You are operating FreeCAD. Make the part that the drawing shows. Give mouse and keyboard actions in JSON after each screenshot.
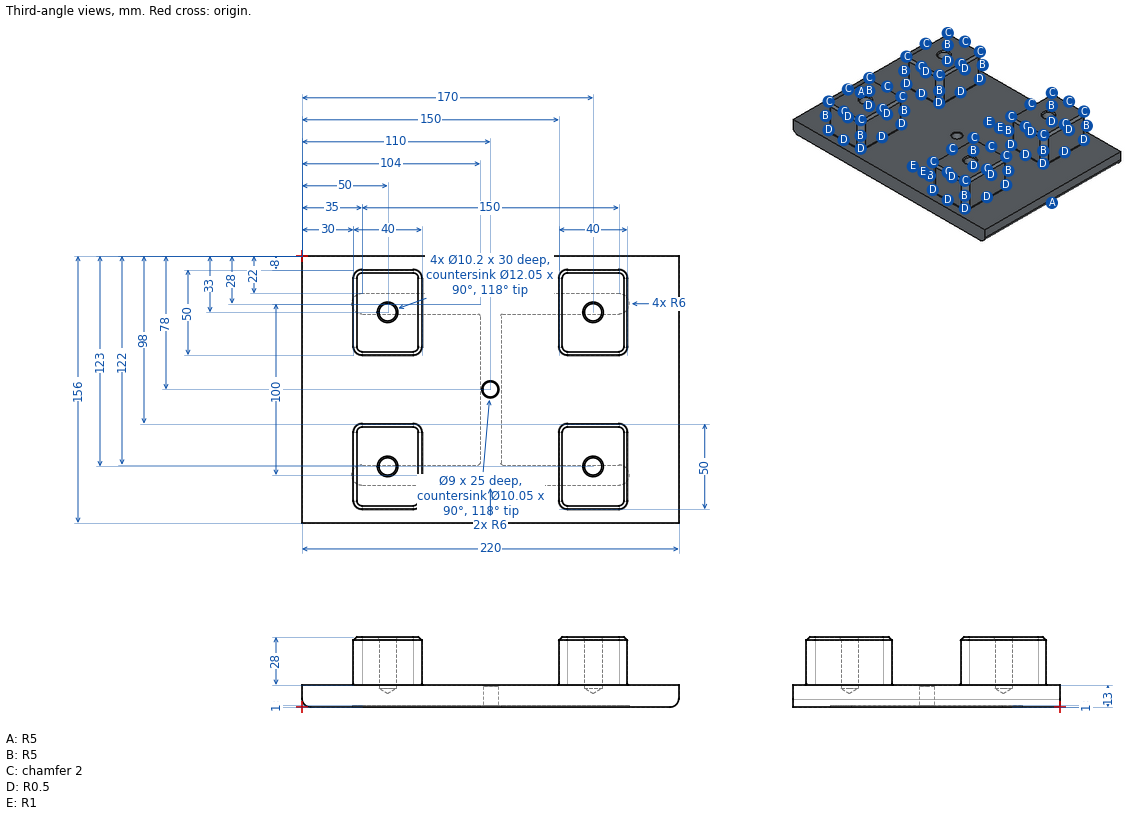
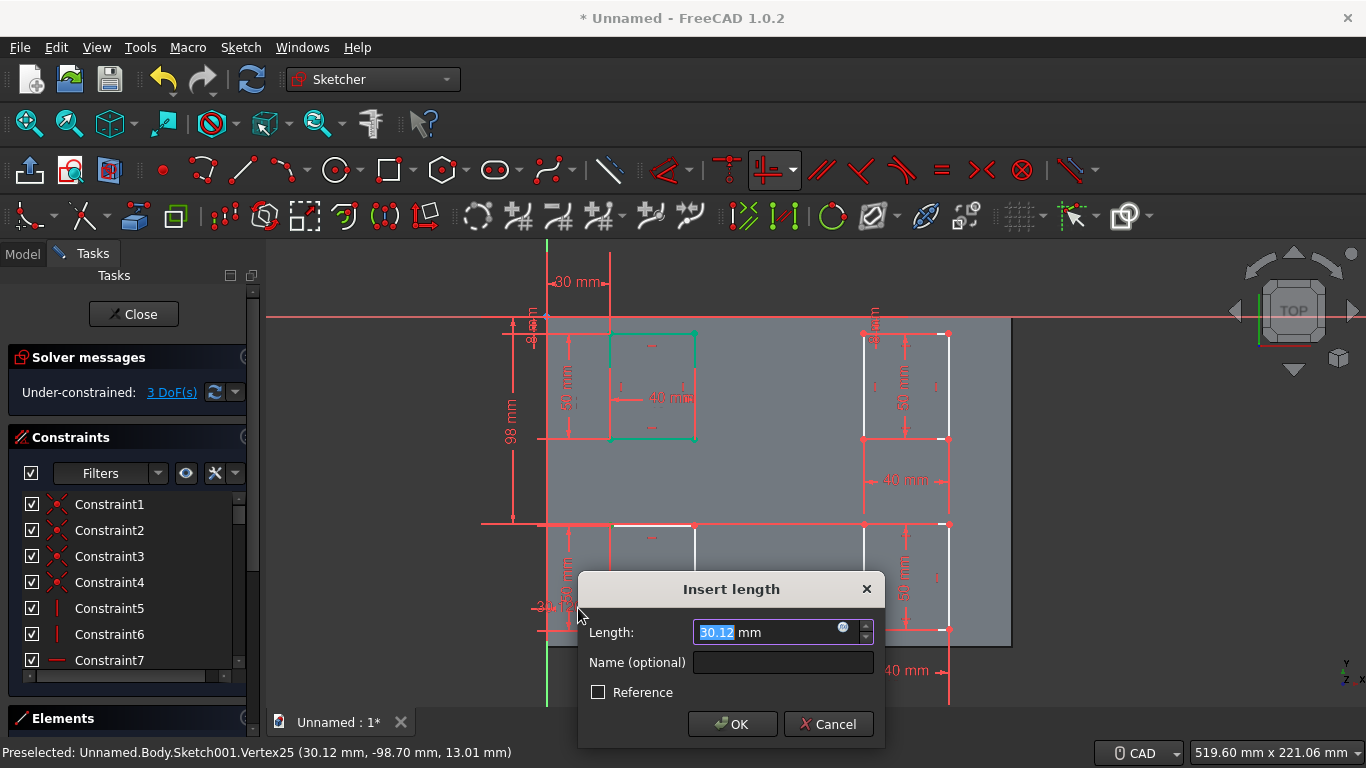
{"action": "type", "text": "30"}
{"action": "key", "text": "Return"}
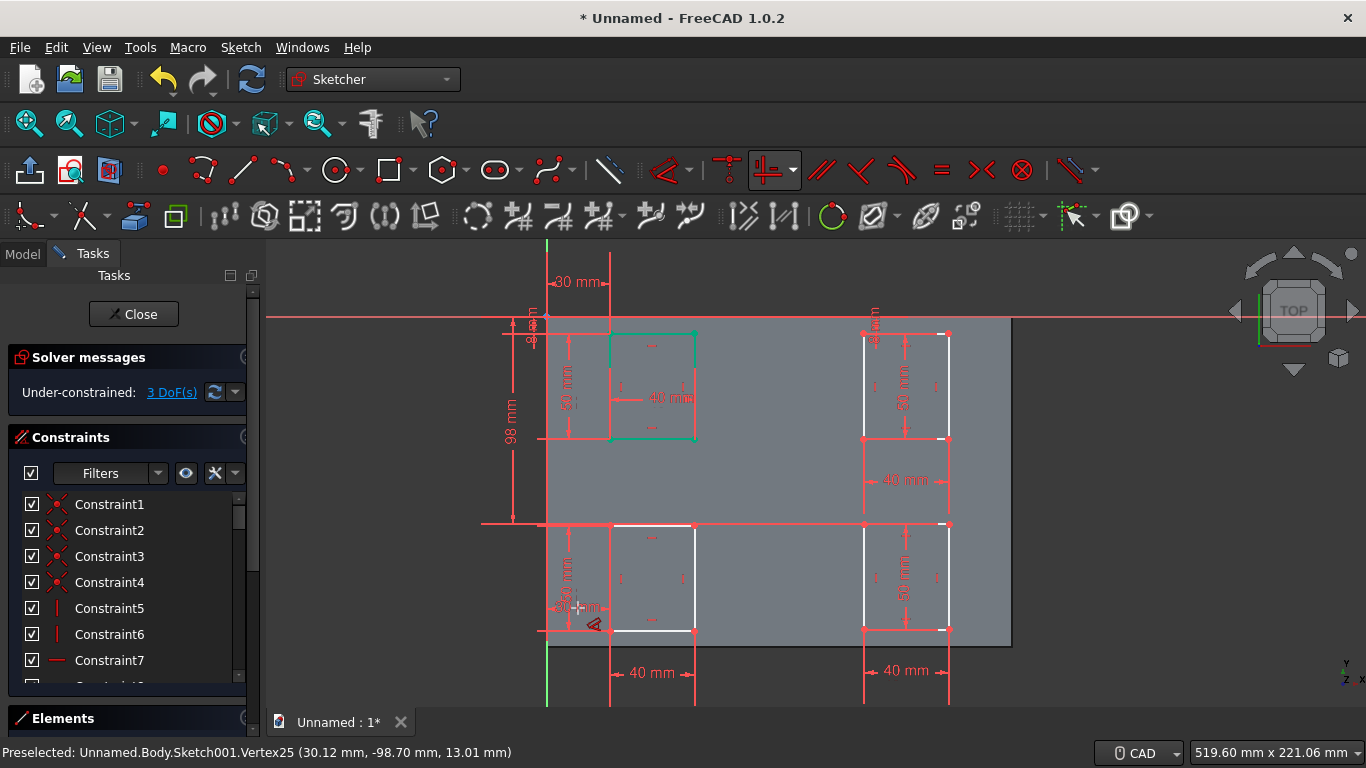
{"action": "left_click", "coordinate": [610, 526]}
{"action": "left_click", "coordinate": [513, 469]}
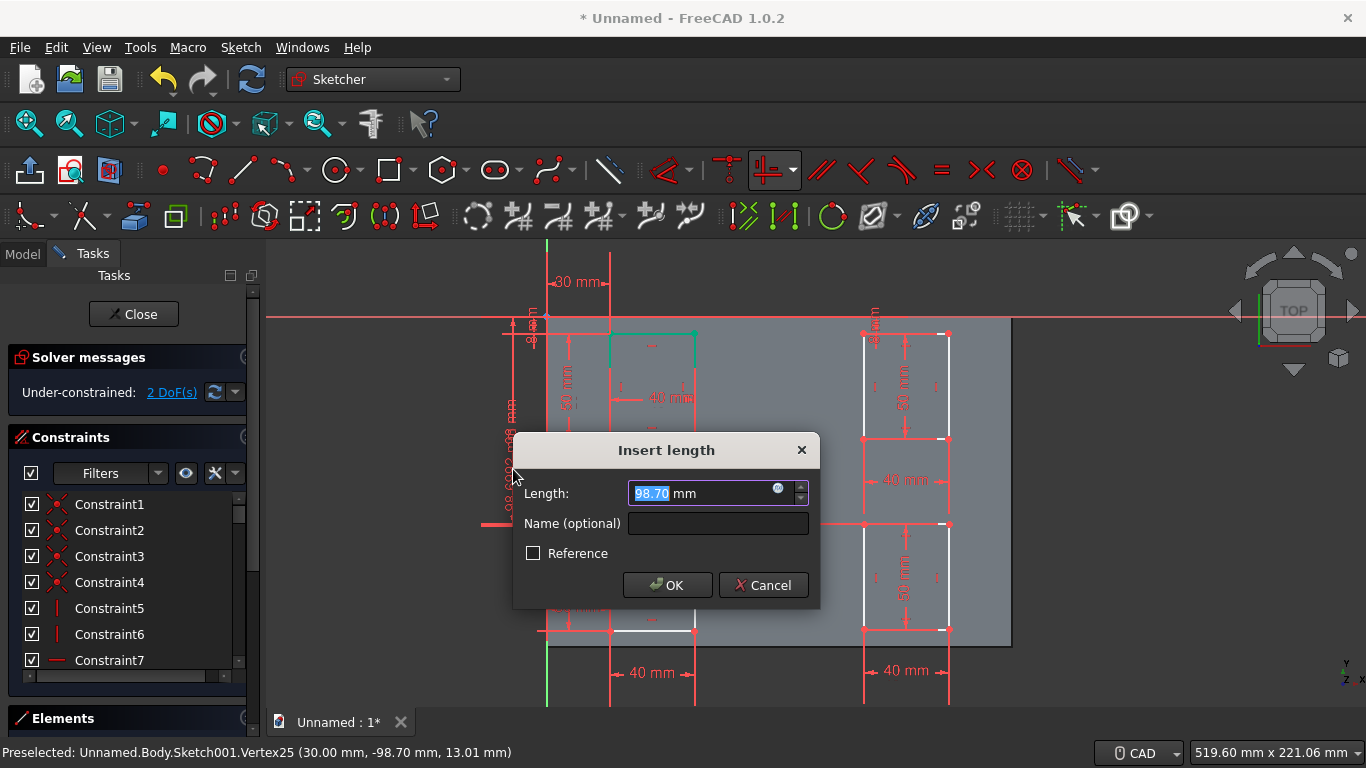
{"action": "type", "text": "98"}
{"action": "key", "text": "Return"}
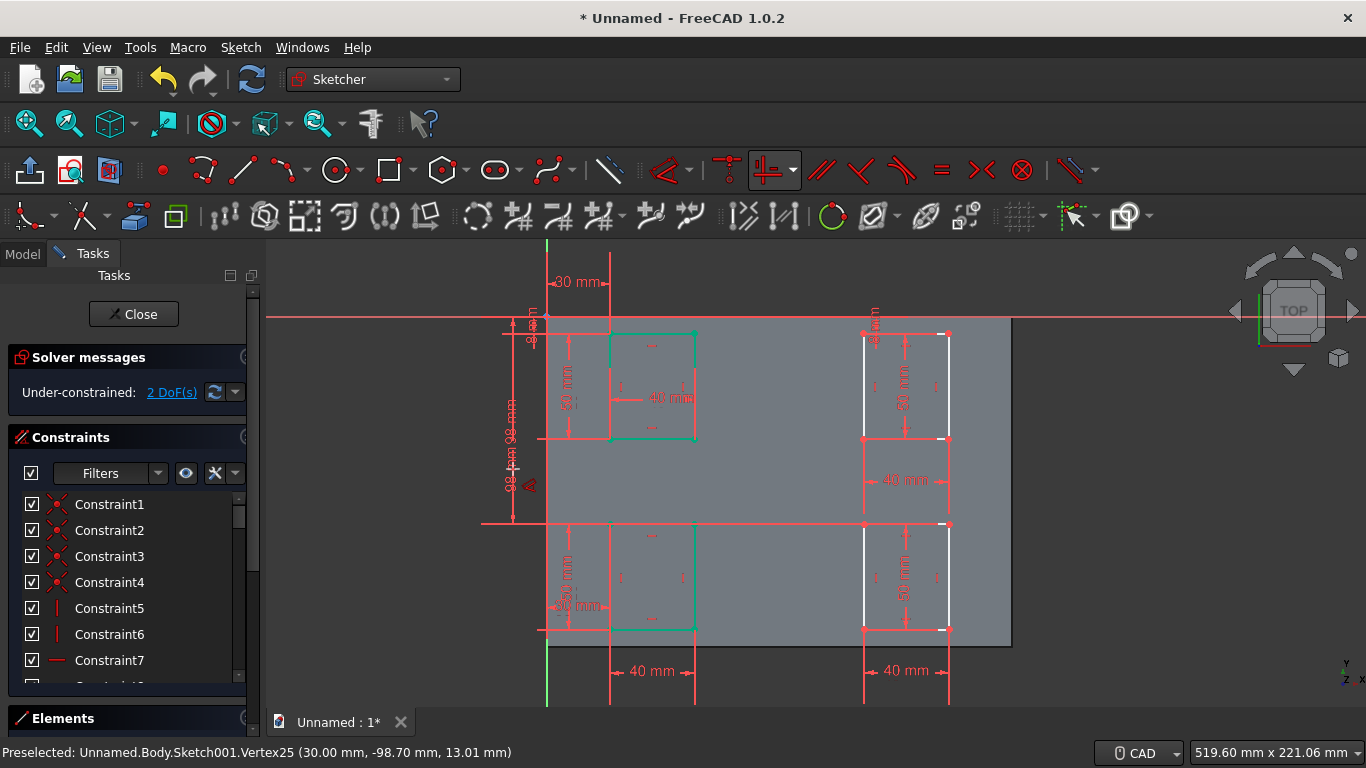
{"action": "left_click", "coordinate": [864, 334]}
{"action": "left_click", "coordinate": [705, 283]}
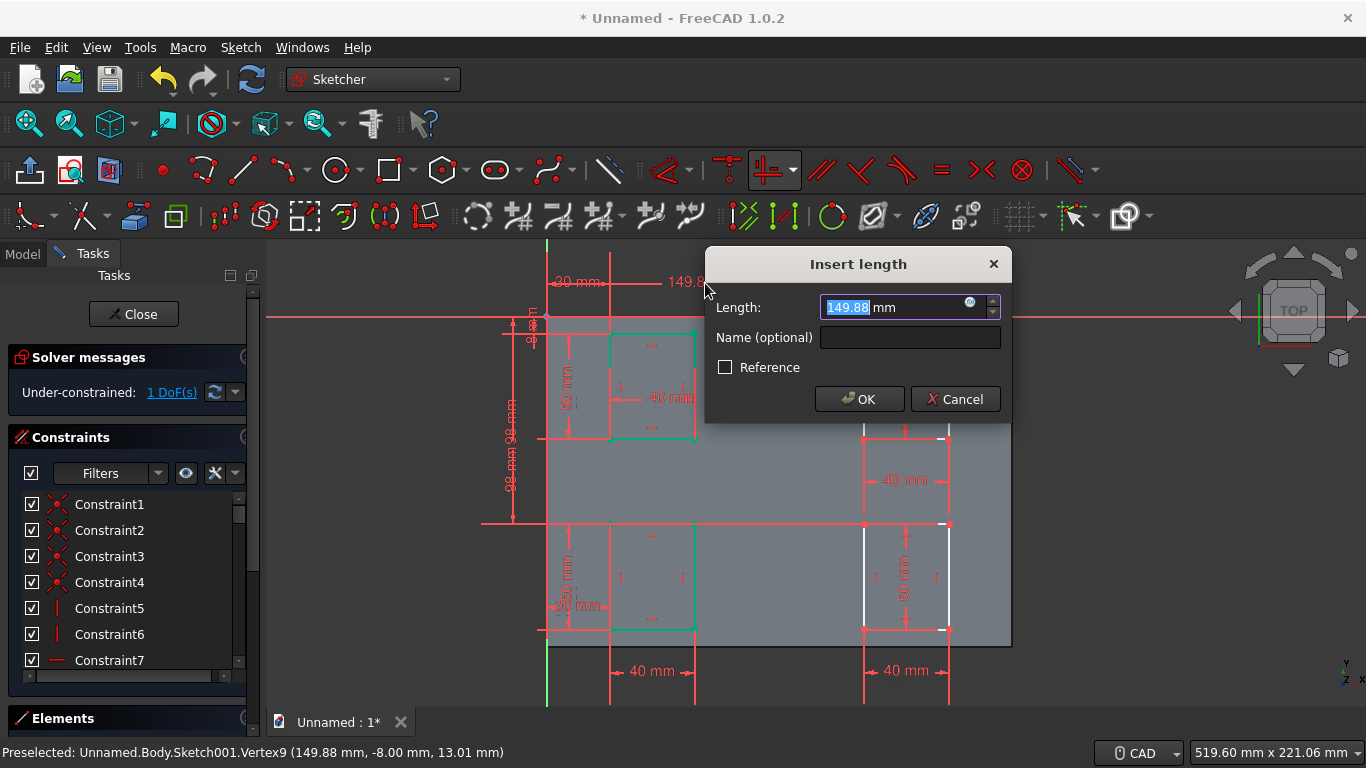
{"action": "type", "text": "150"}
{"action": "key", "text": "Return"}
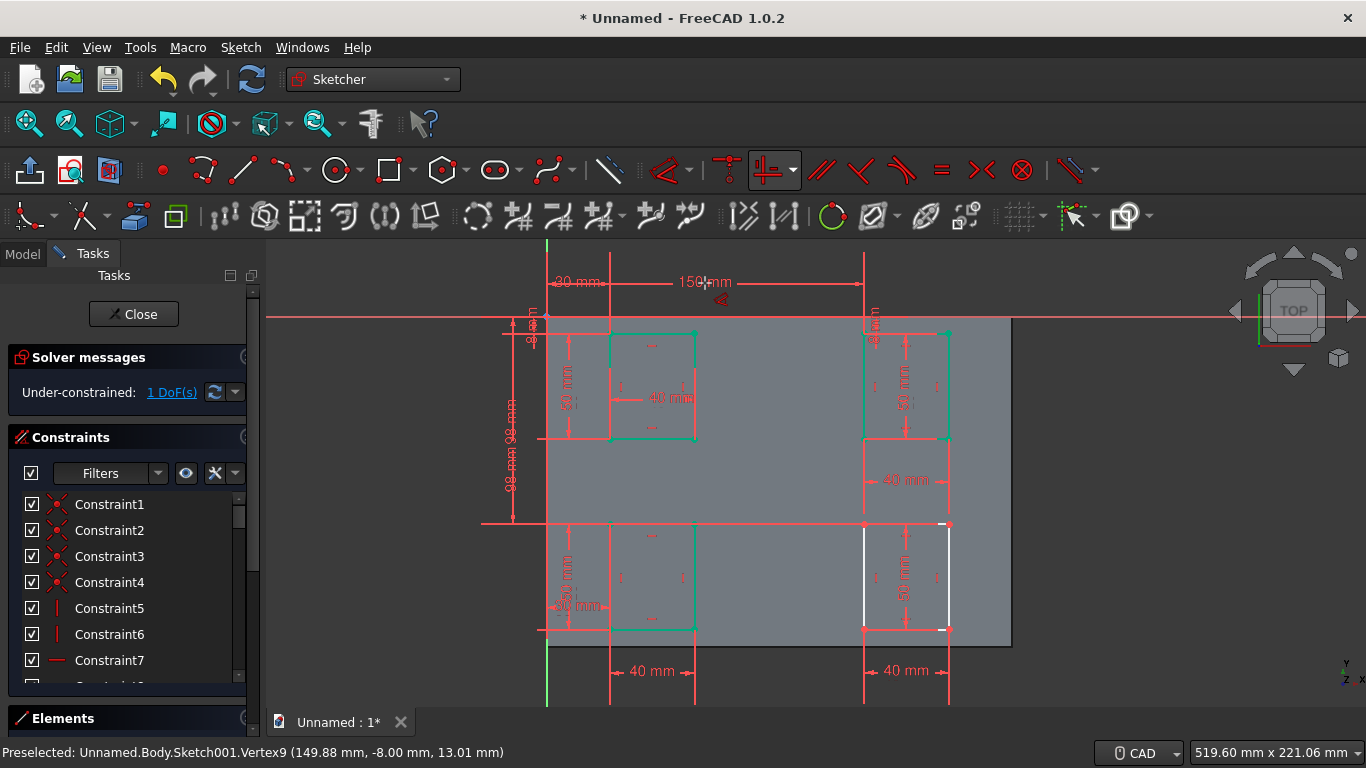
{"action": "left_click", "coordinate": [864, 524]}
{"action": "left_click", "coordinate": [779, 283]}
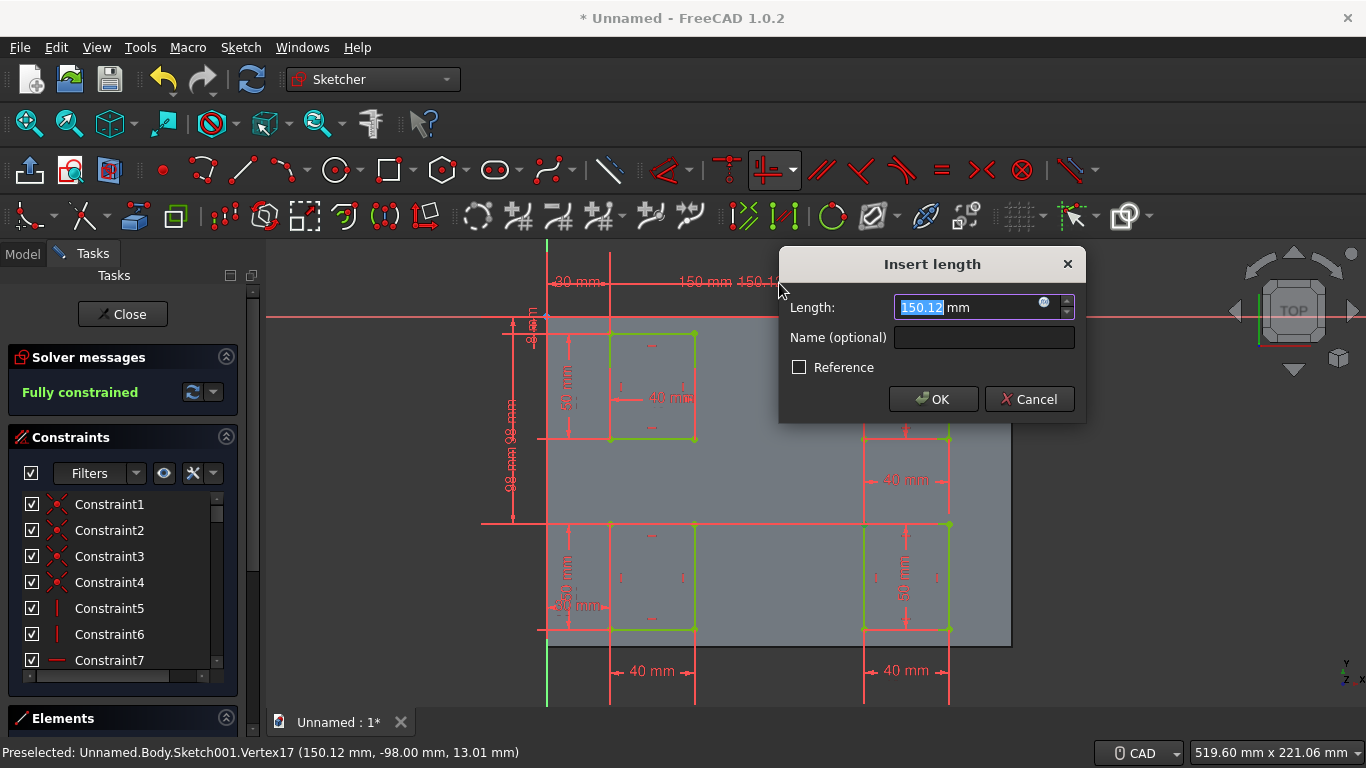
{"action": "type", "text": "150"}
{"action": "key", "text": "Return"}
{"action": "key", "text": "Escape"}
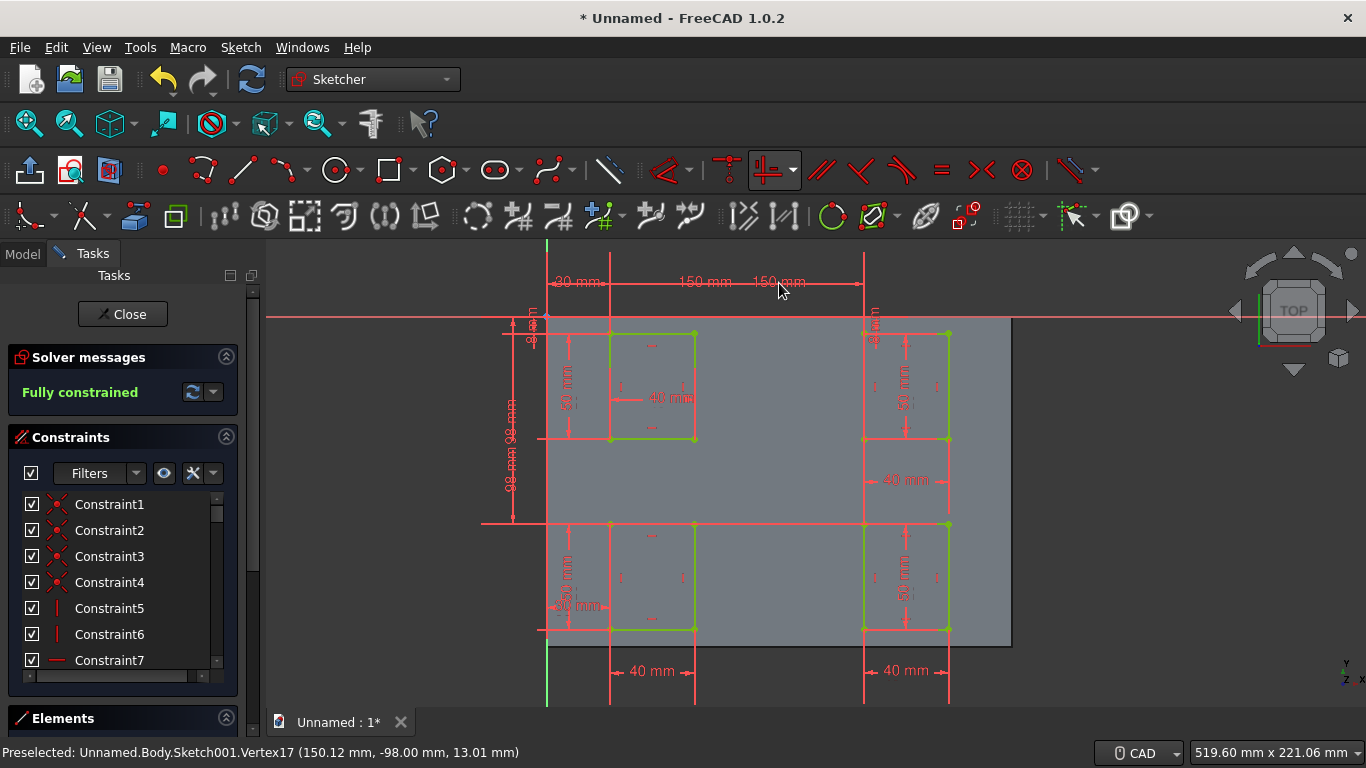
{"action": "left_click", "coordinate": [123, 314]}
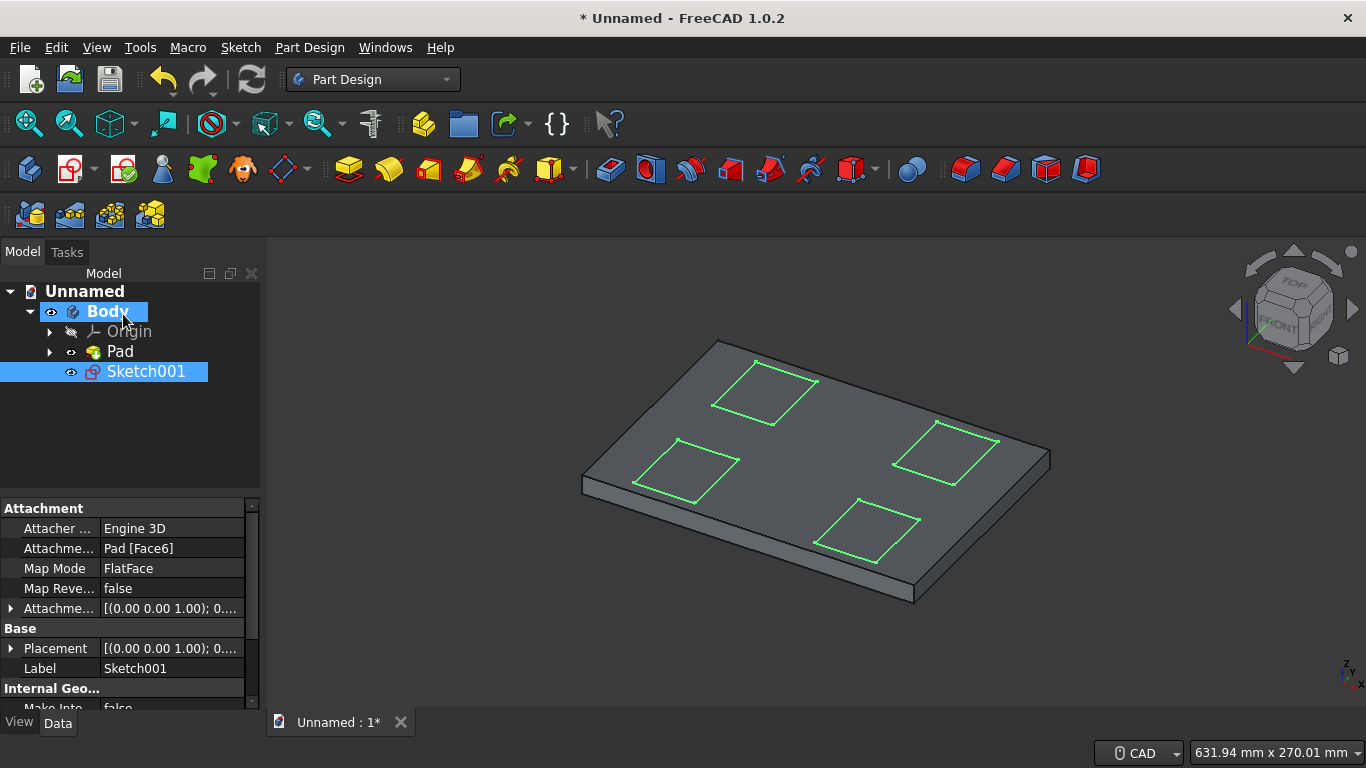
{"action": "left_click", "coordinate": [350, 170]}